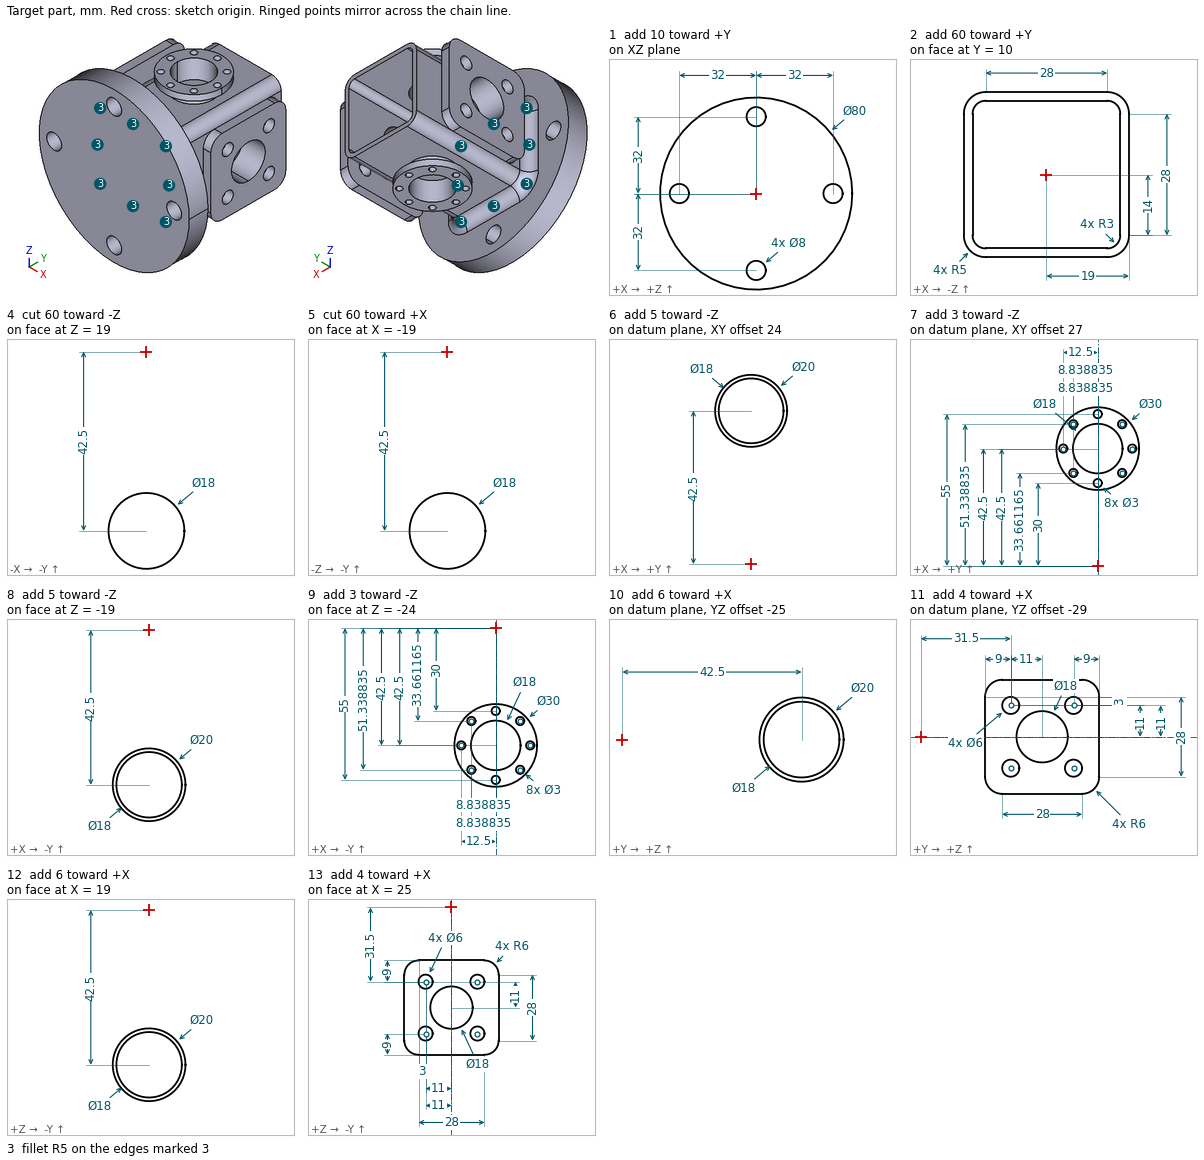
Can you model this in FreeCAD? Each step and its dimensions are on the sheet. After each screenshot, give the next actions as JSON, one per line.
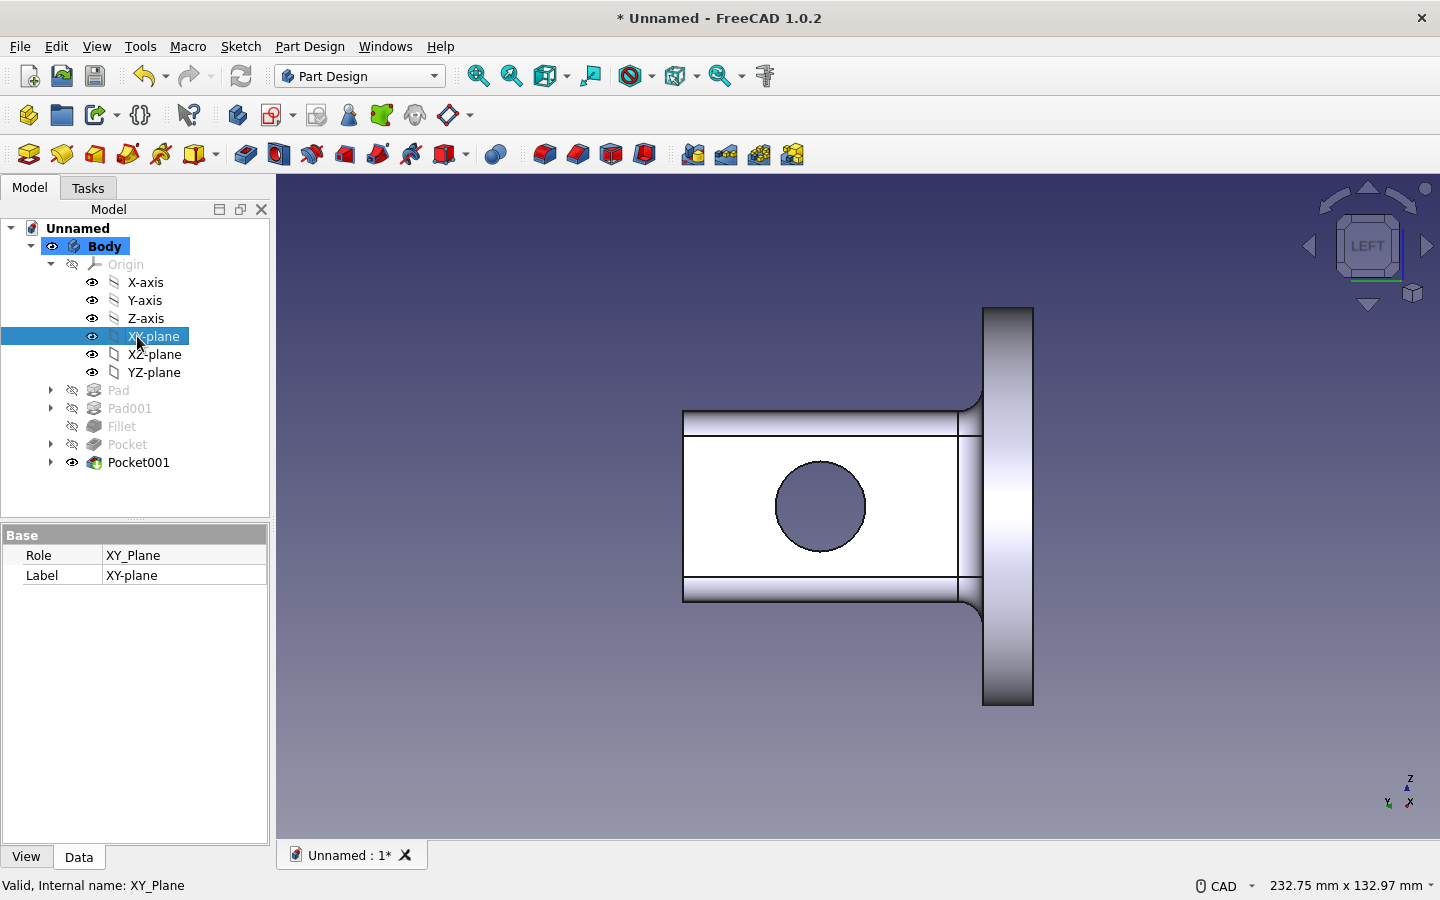
{"action": "left_click", "coordinate": [448, 116]}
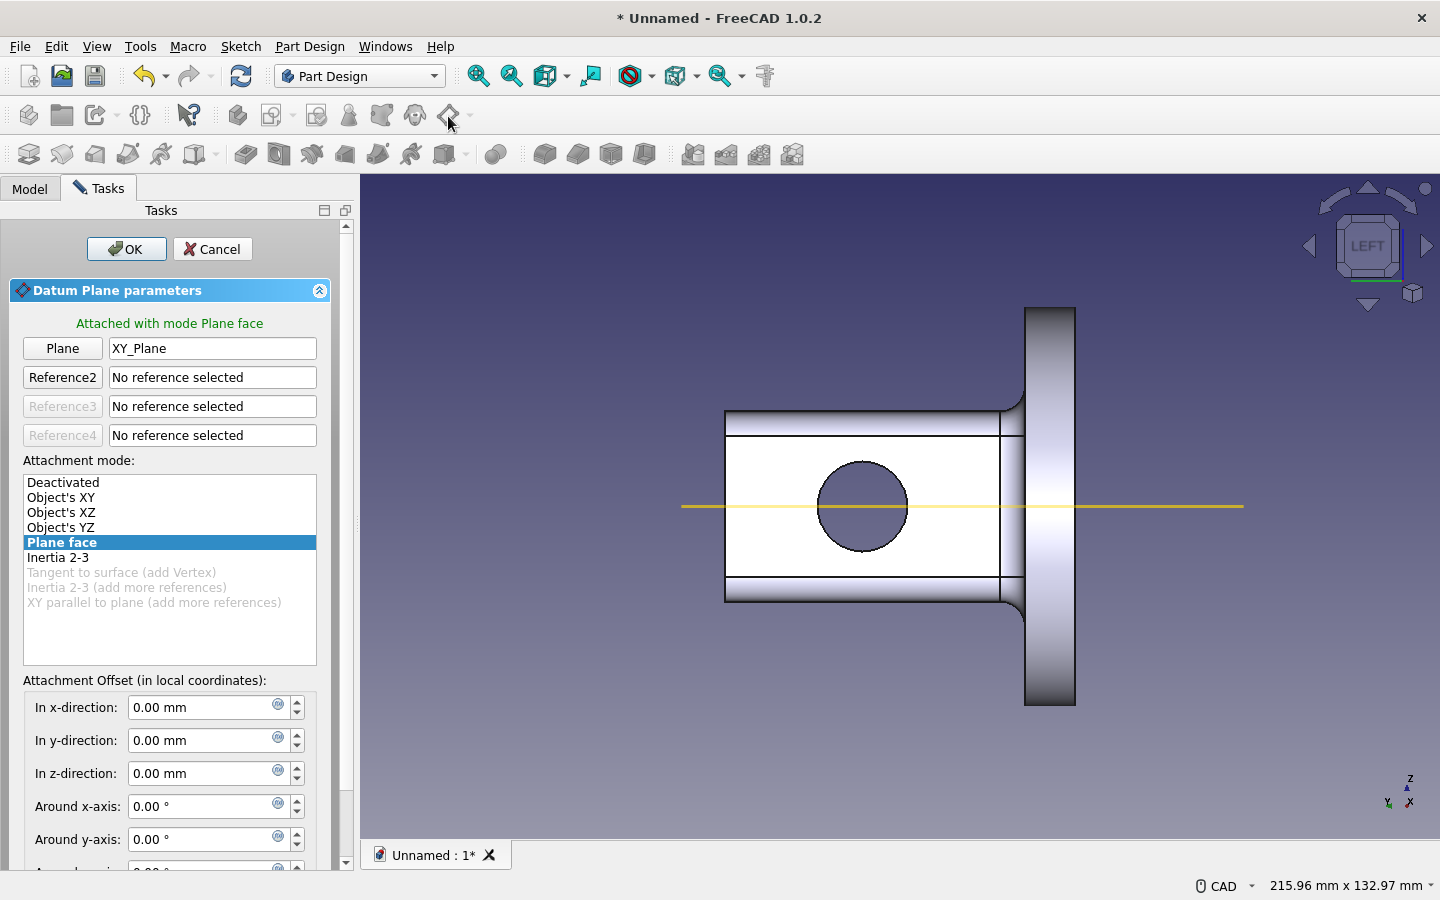
{"action": "triple_click", "coordinate": [210, 774]}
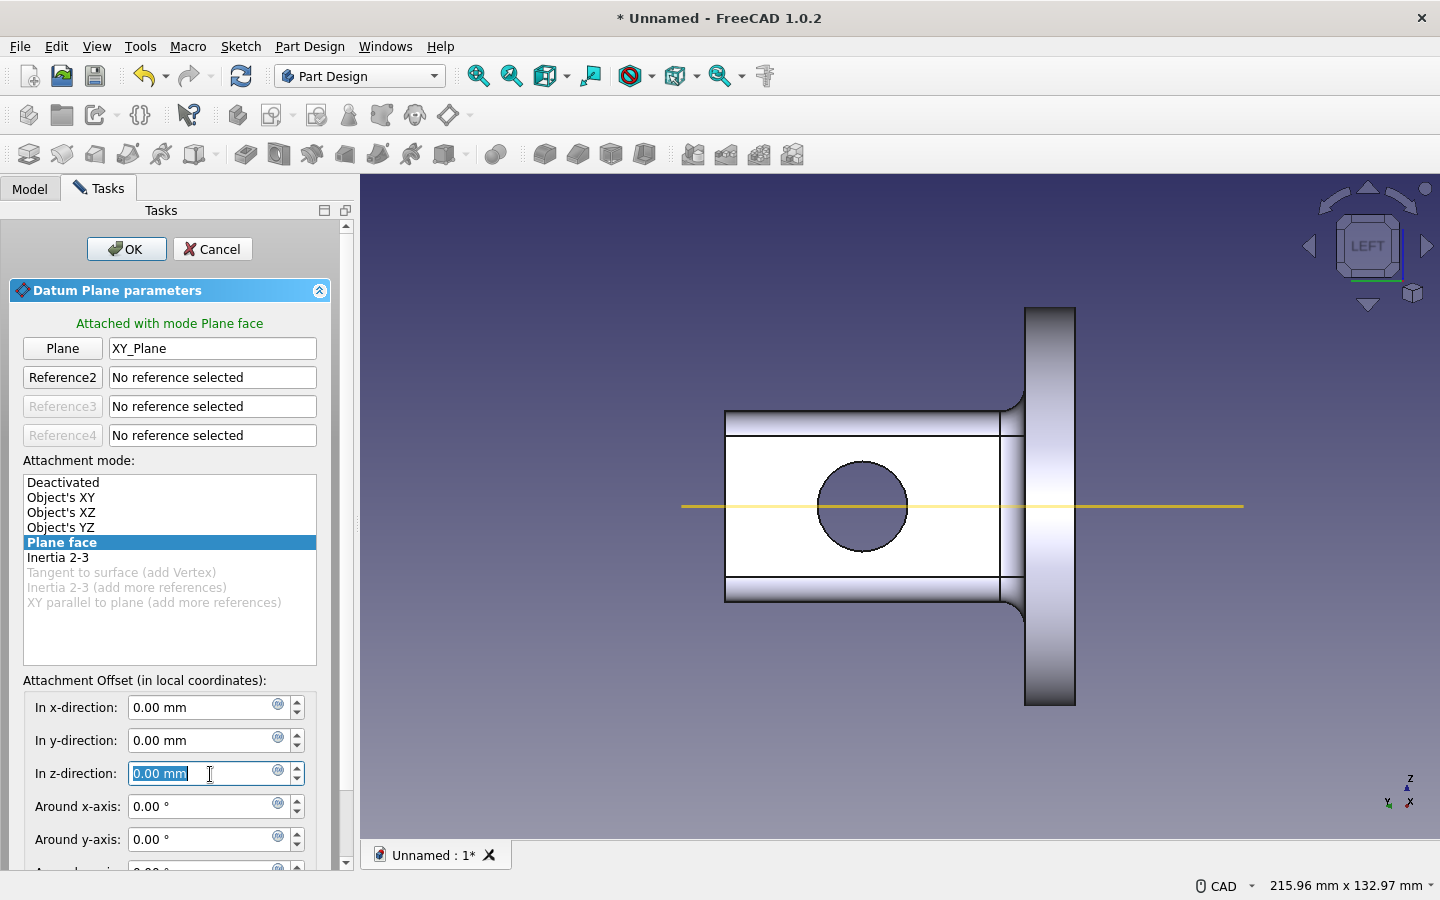
{"action": "type", "text": "24"}
{"action": "key", "text": "Tab"}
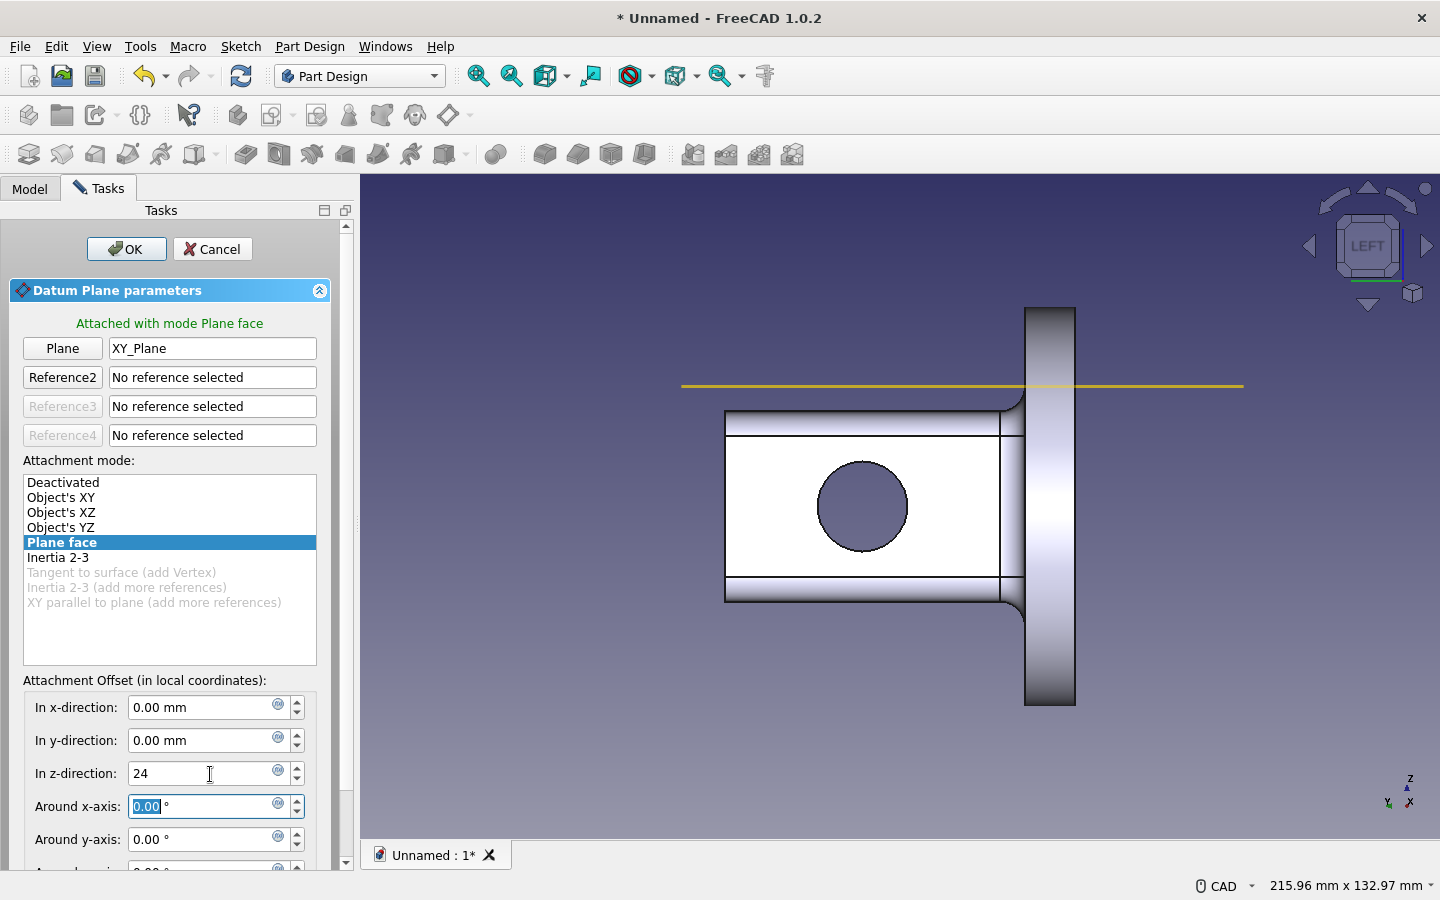
{"action": "left_click", "coordinate": [127, 249]}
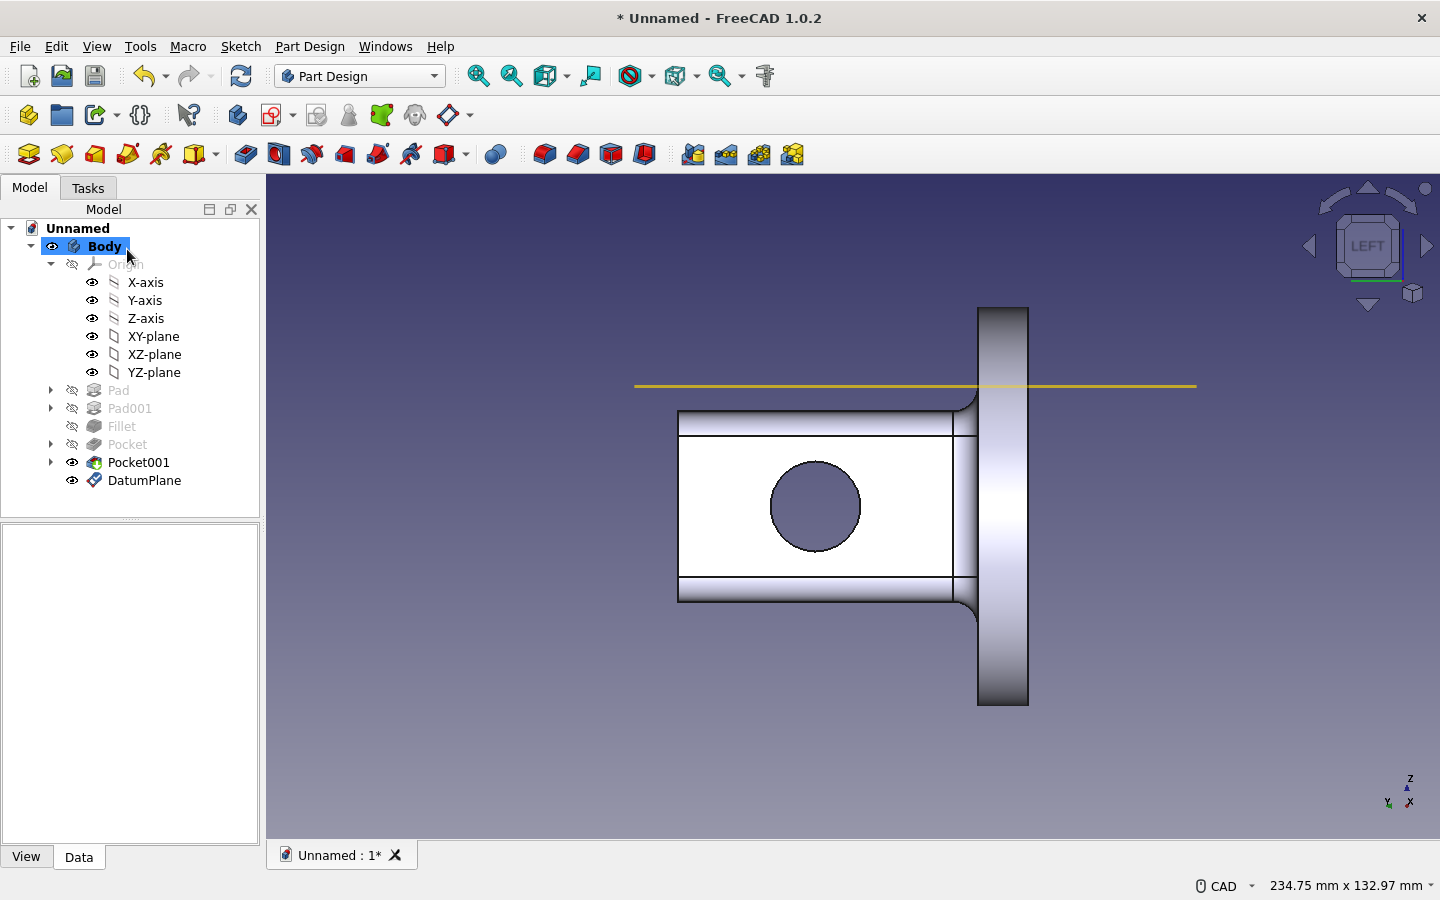
{"action": "left_click", "coordinate": [117, 480]}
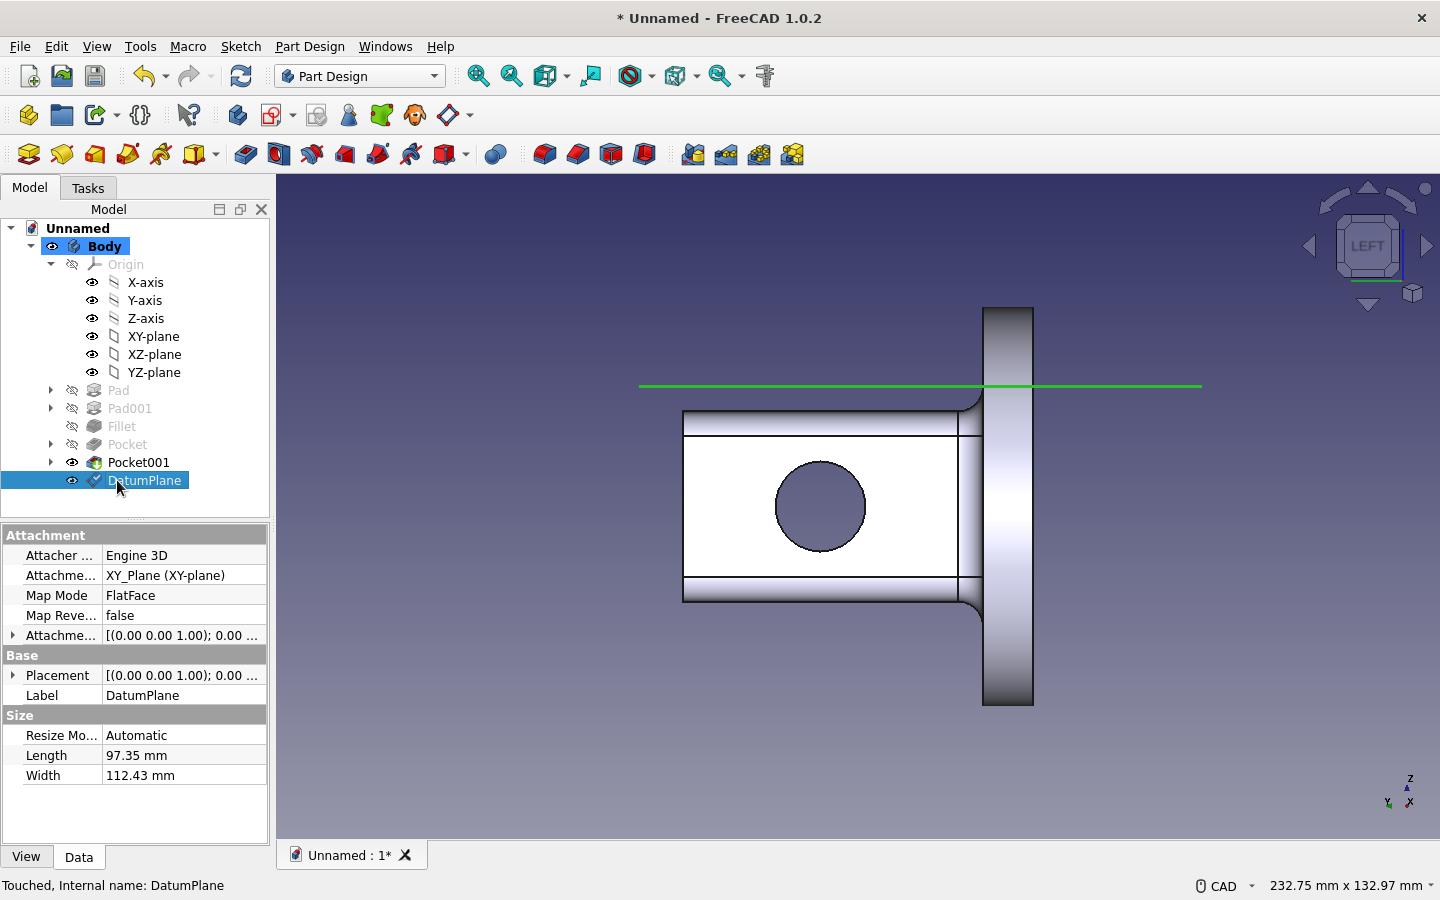
{"action": "left_click", "coordinate": [270, 116]}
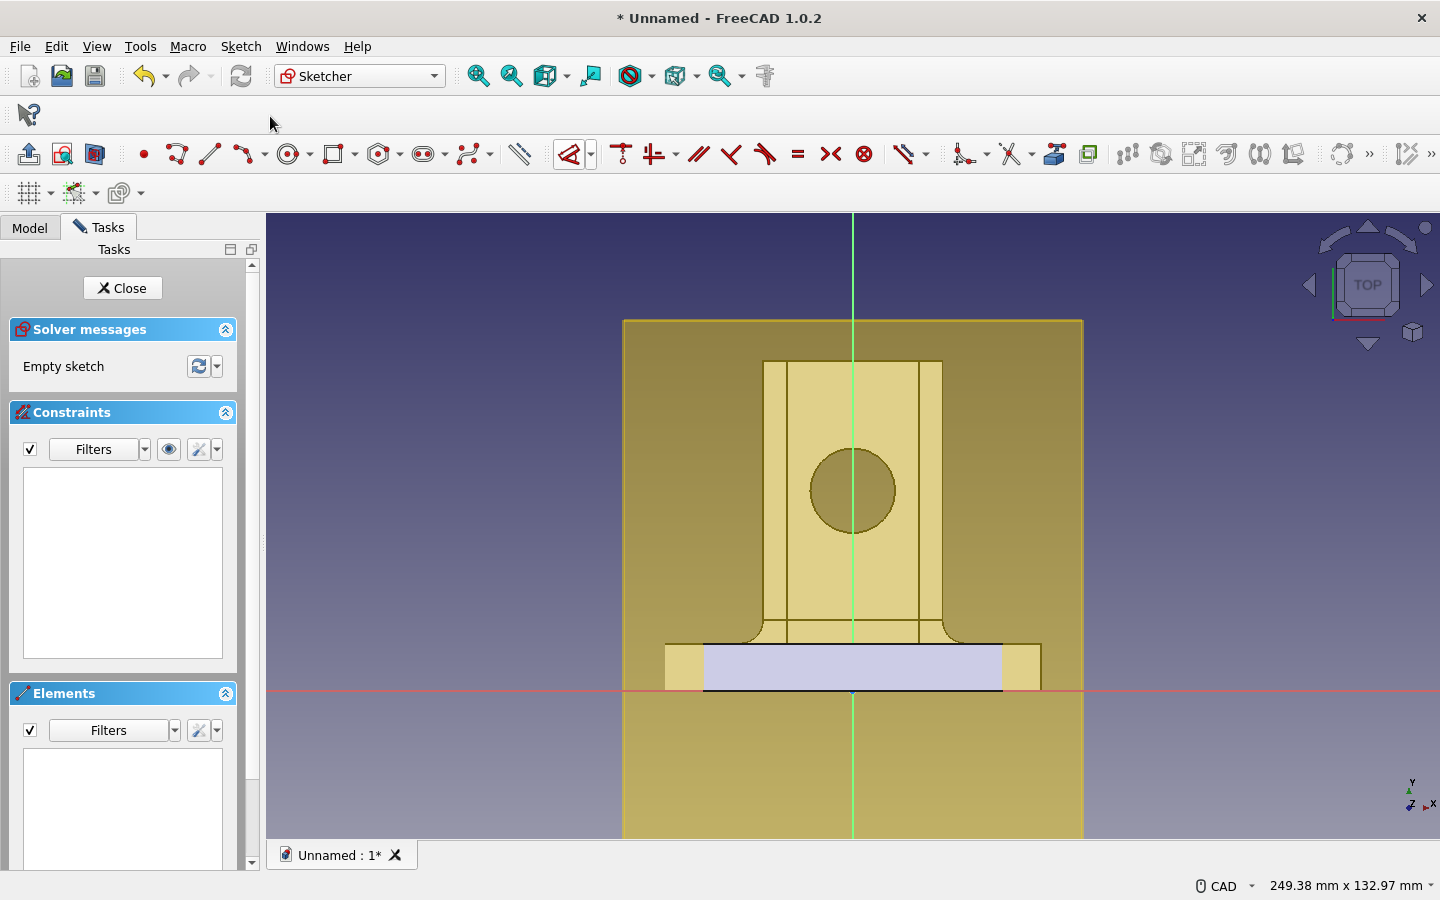
{"action": "key", "text": "q s"}